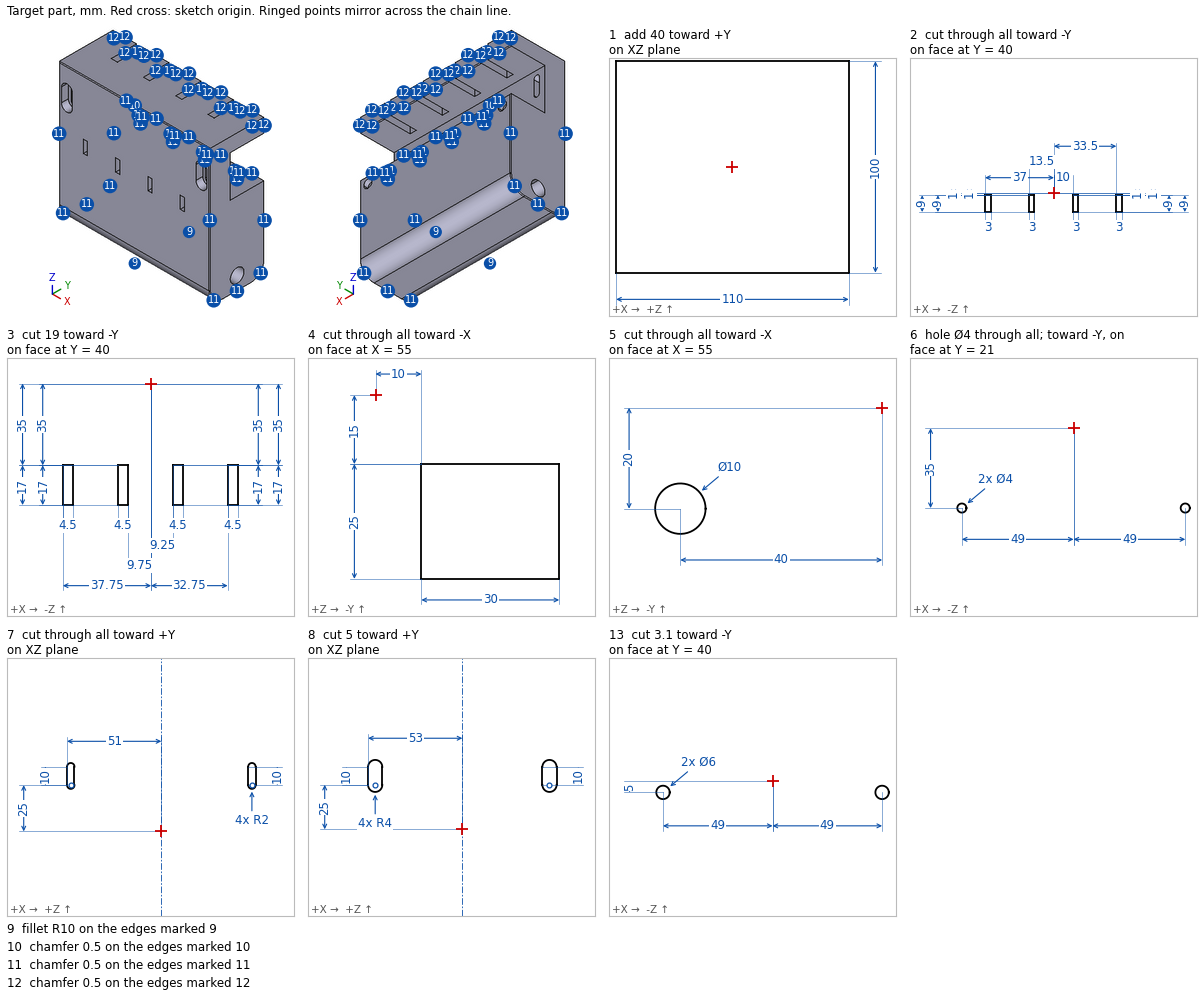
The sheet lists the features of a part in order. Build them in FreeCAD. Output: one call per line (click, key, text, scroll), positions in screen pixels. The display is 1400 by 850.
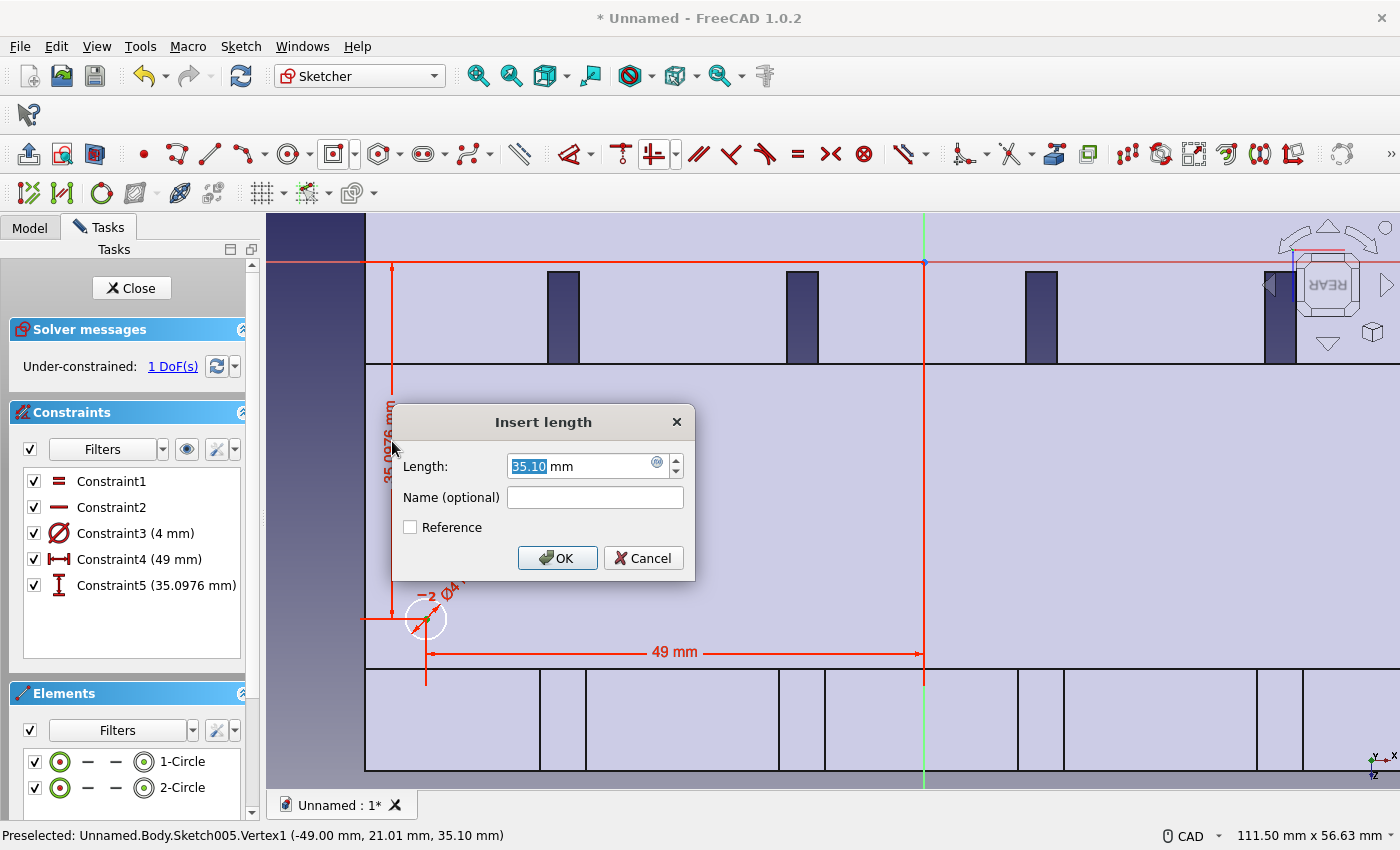
text(35)
key(Return)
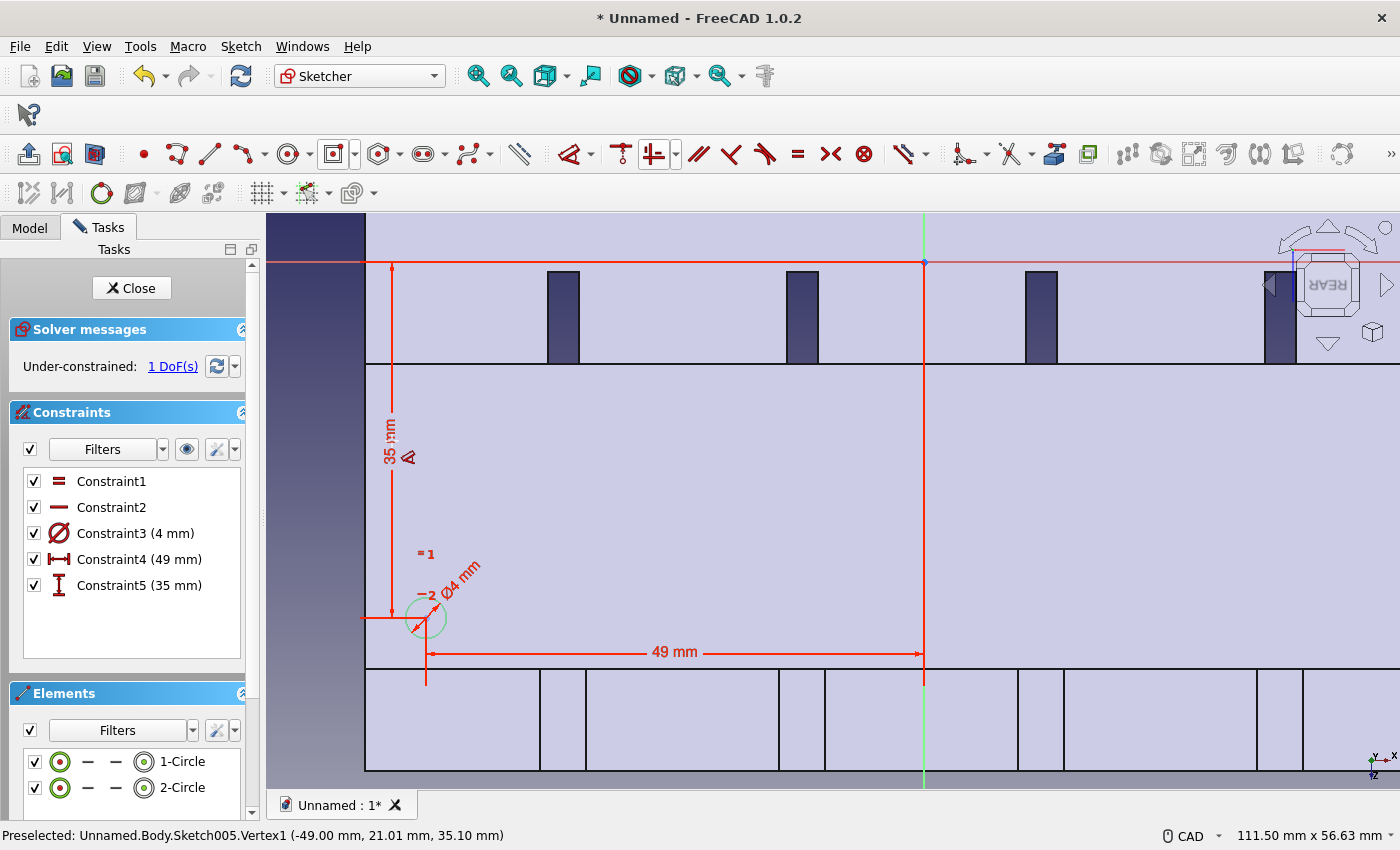
scroll(439, 604, down, 2)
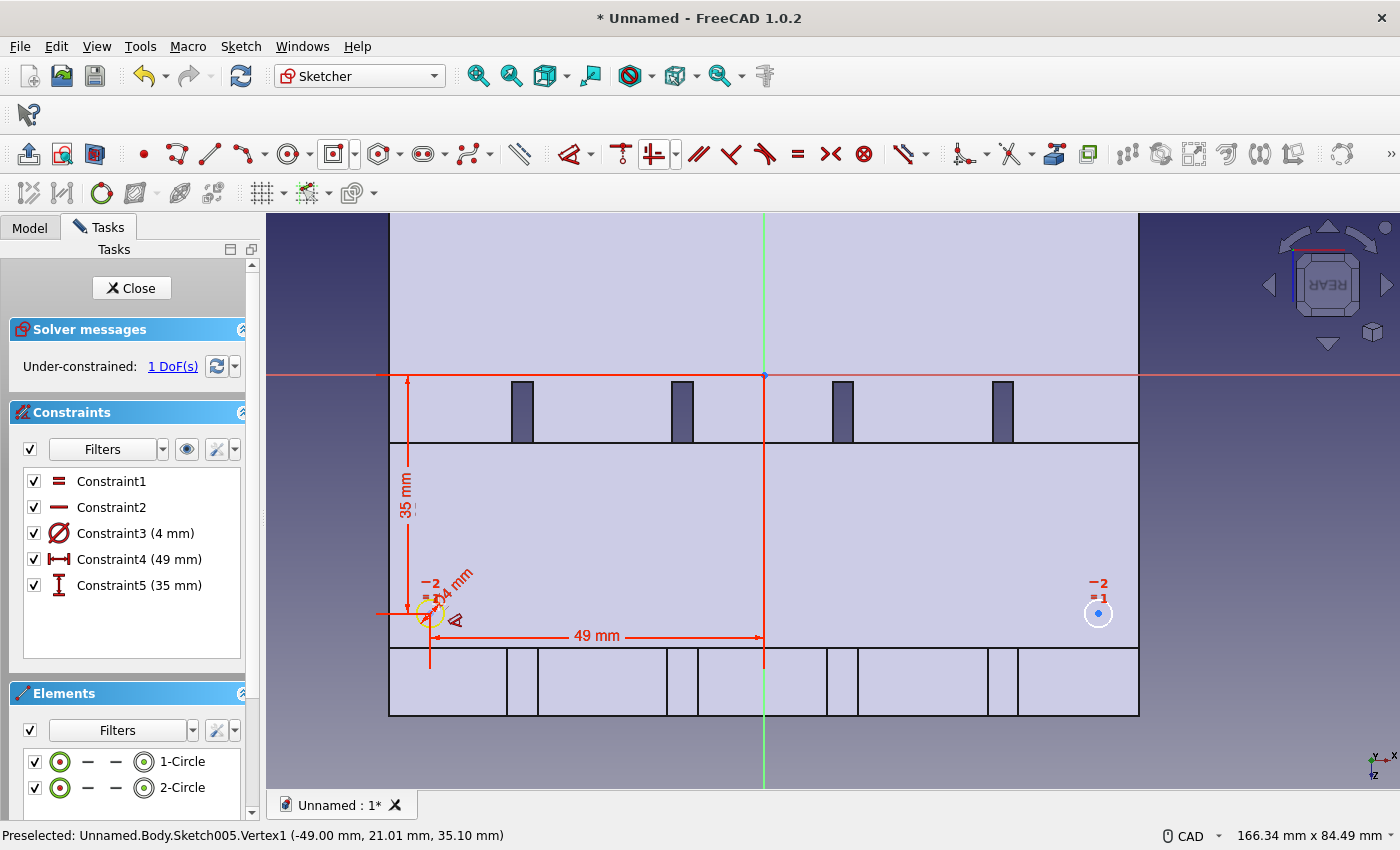
click(1098, 614)
click(931, 341)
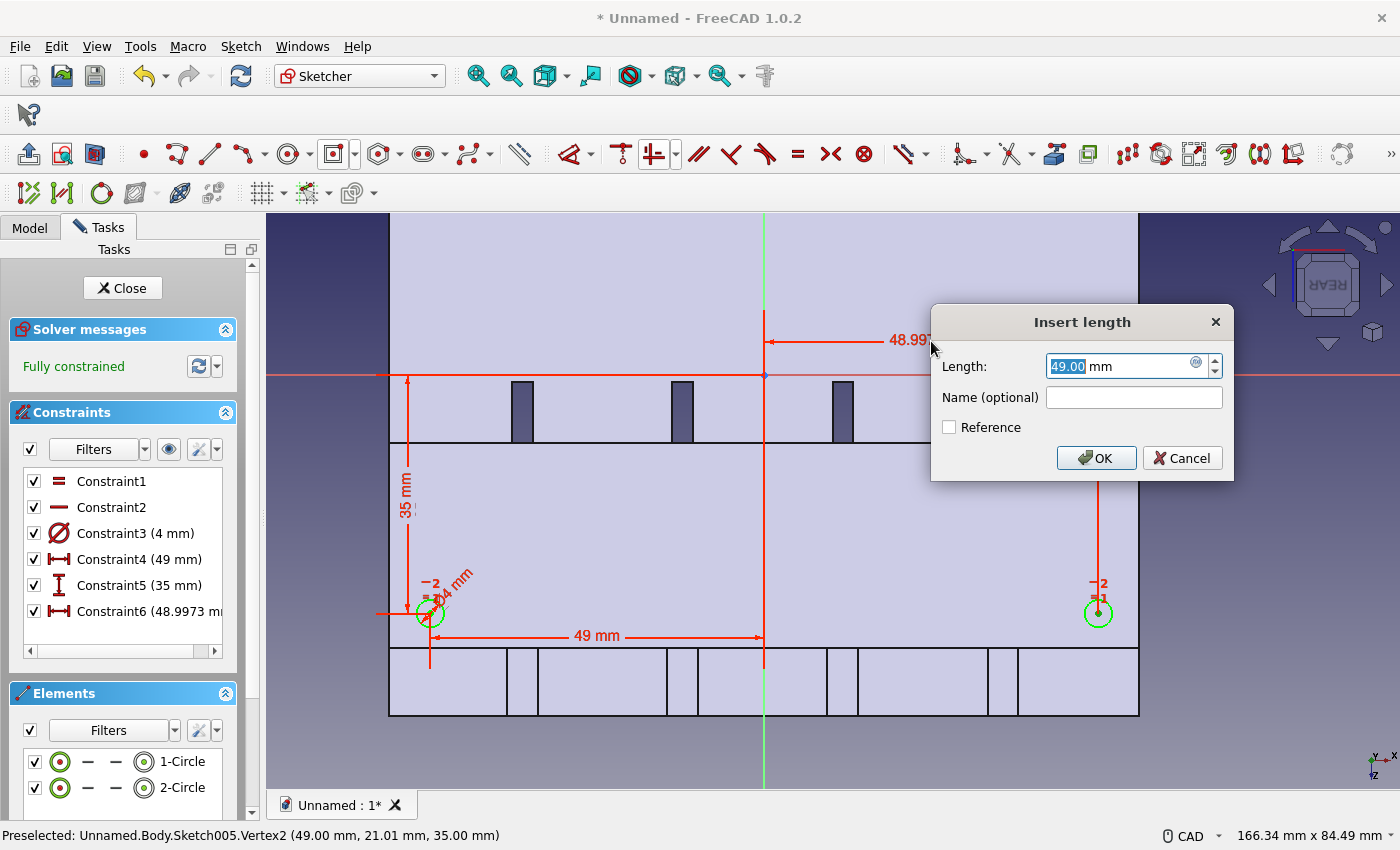
text(49)
key(Return)
key(Escape)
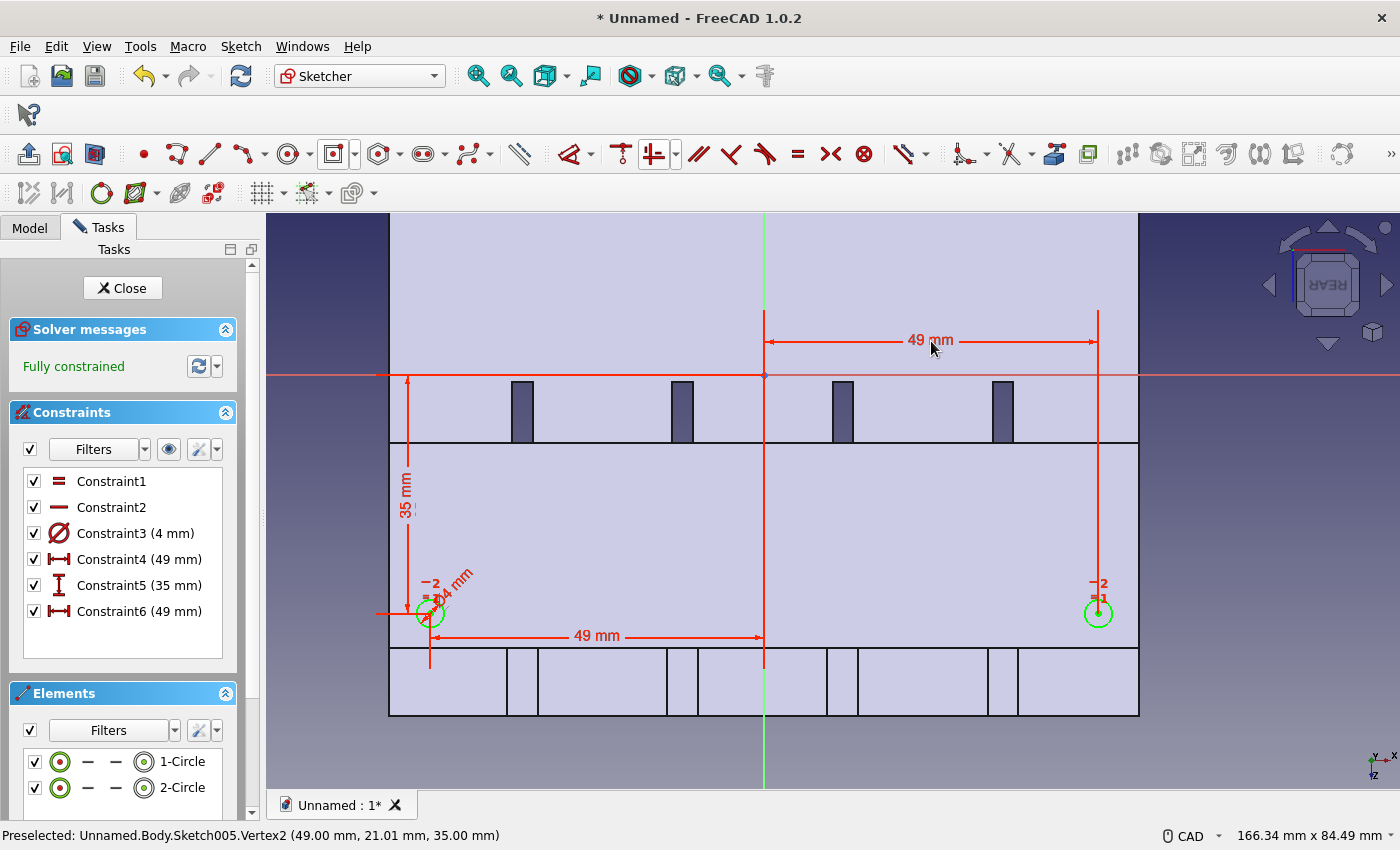
click(123, 288)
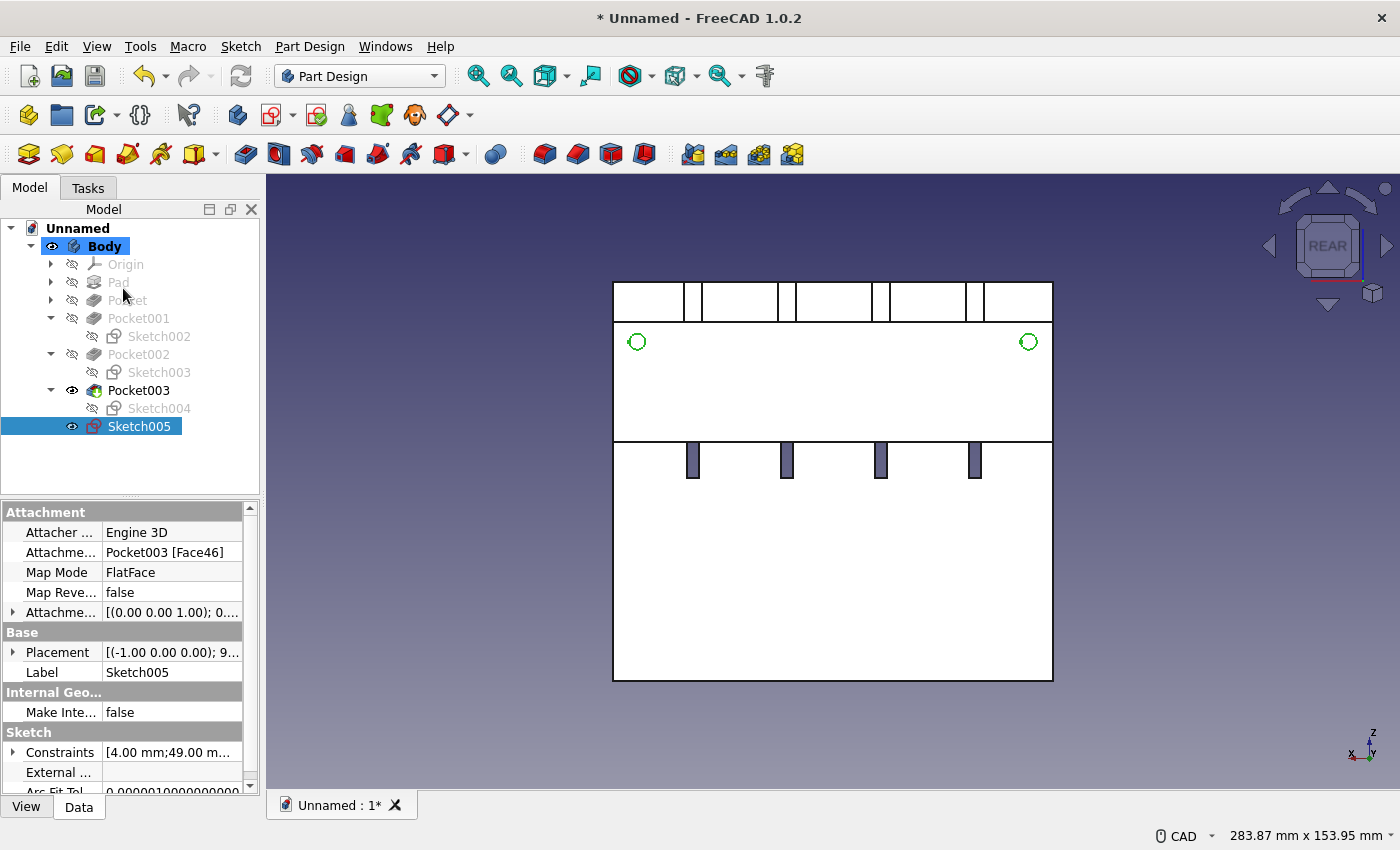
click(279, 154)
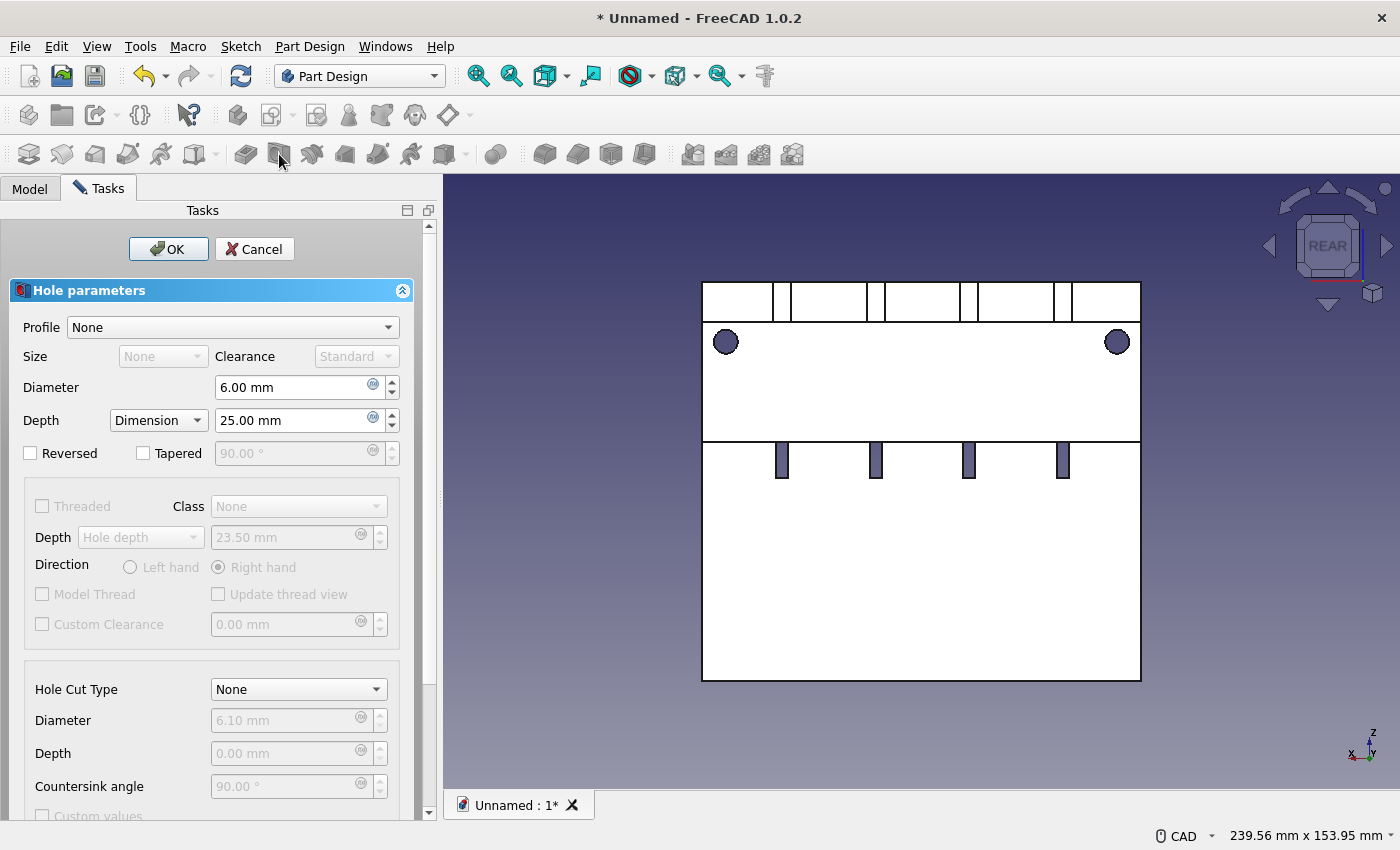
triple_click(300, 388)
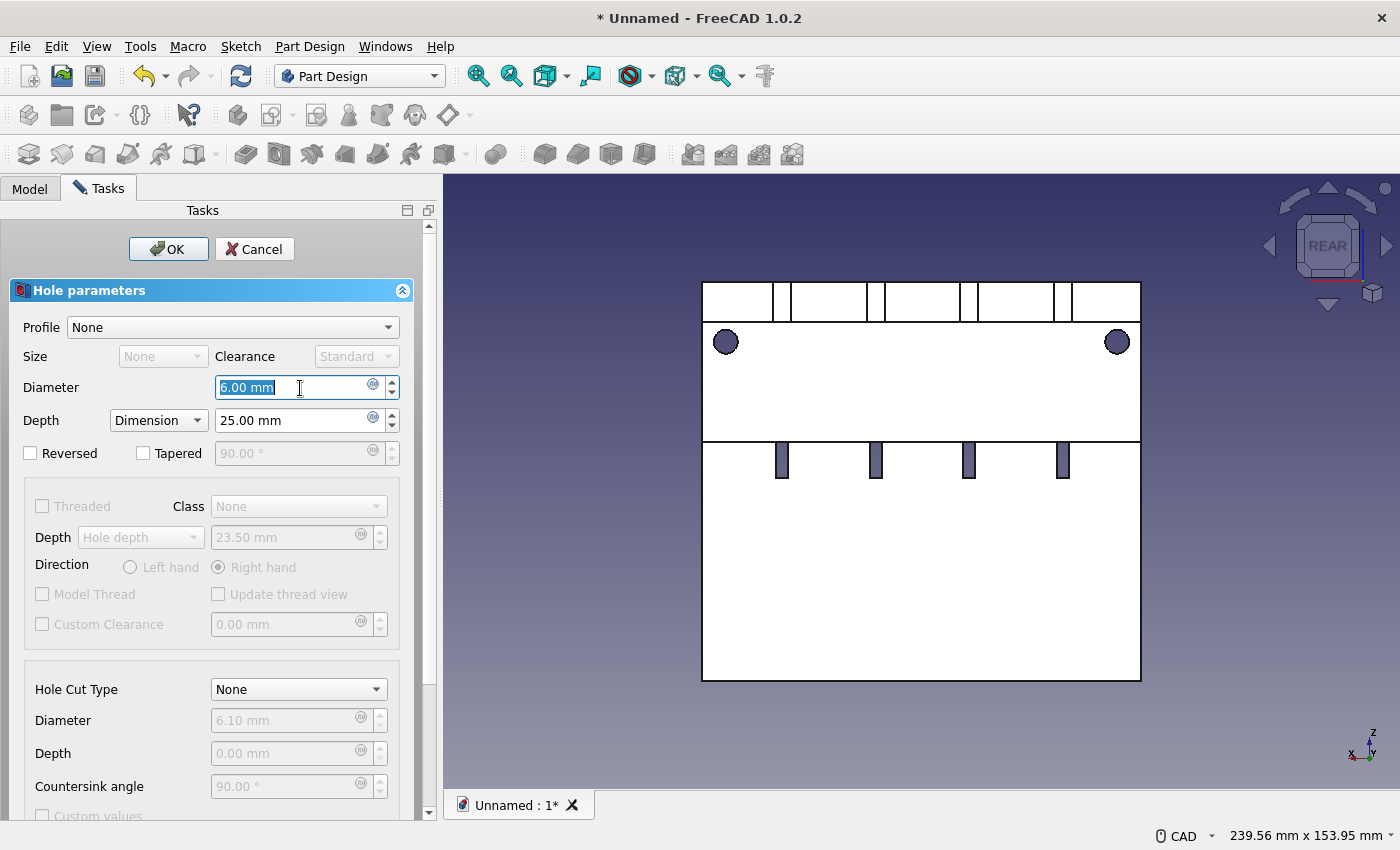
text(4)
key(Tab)